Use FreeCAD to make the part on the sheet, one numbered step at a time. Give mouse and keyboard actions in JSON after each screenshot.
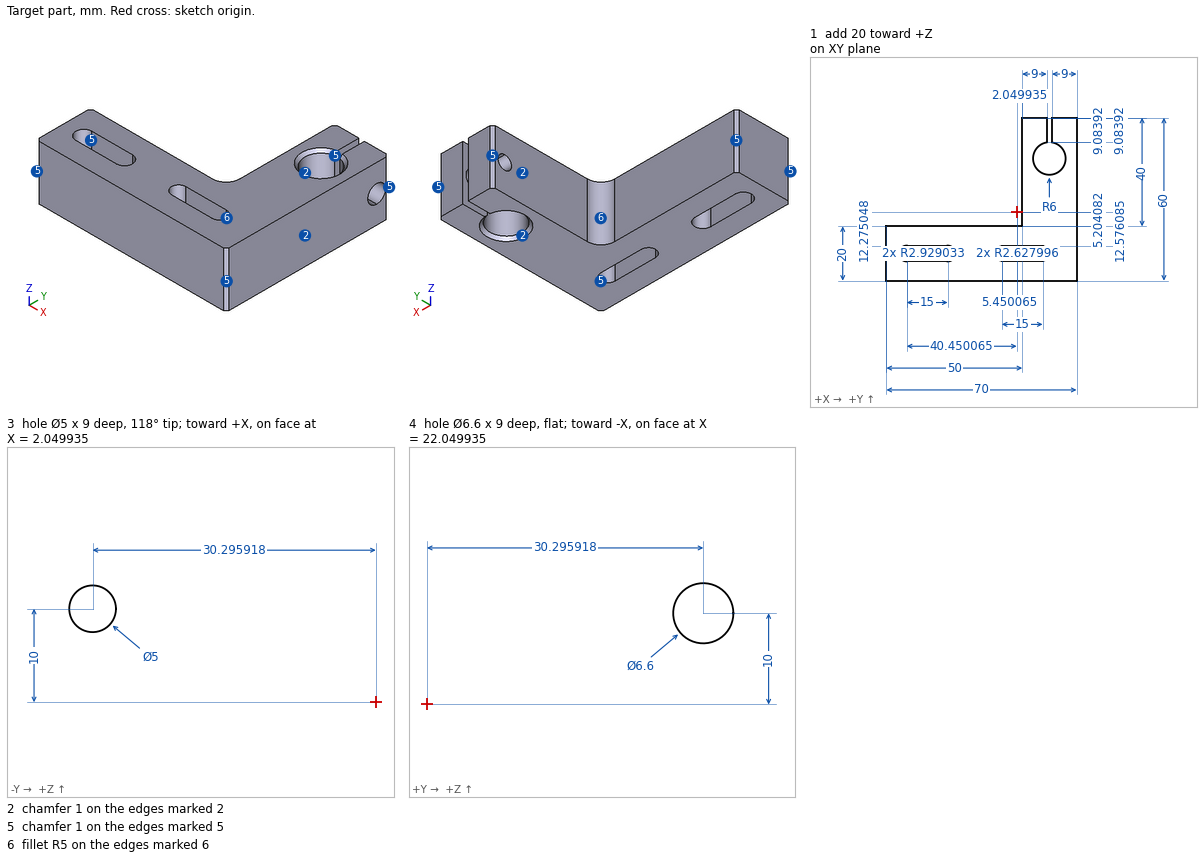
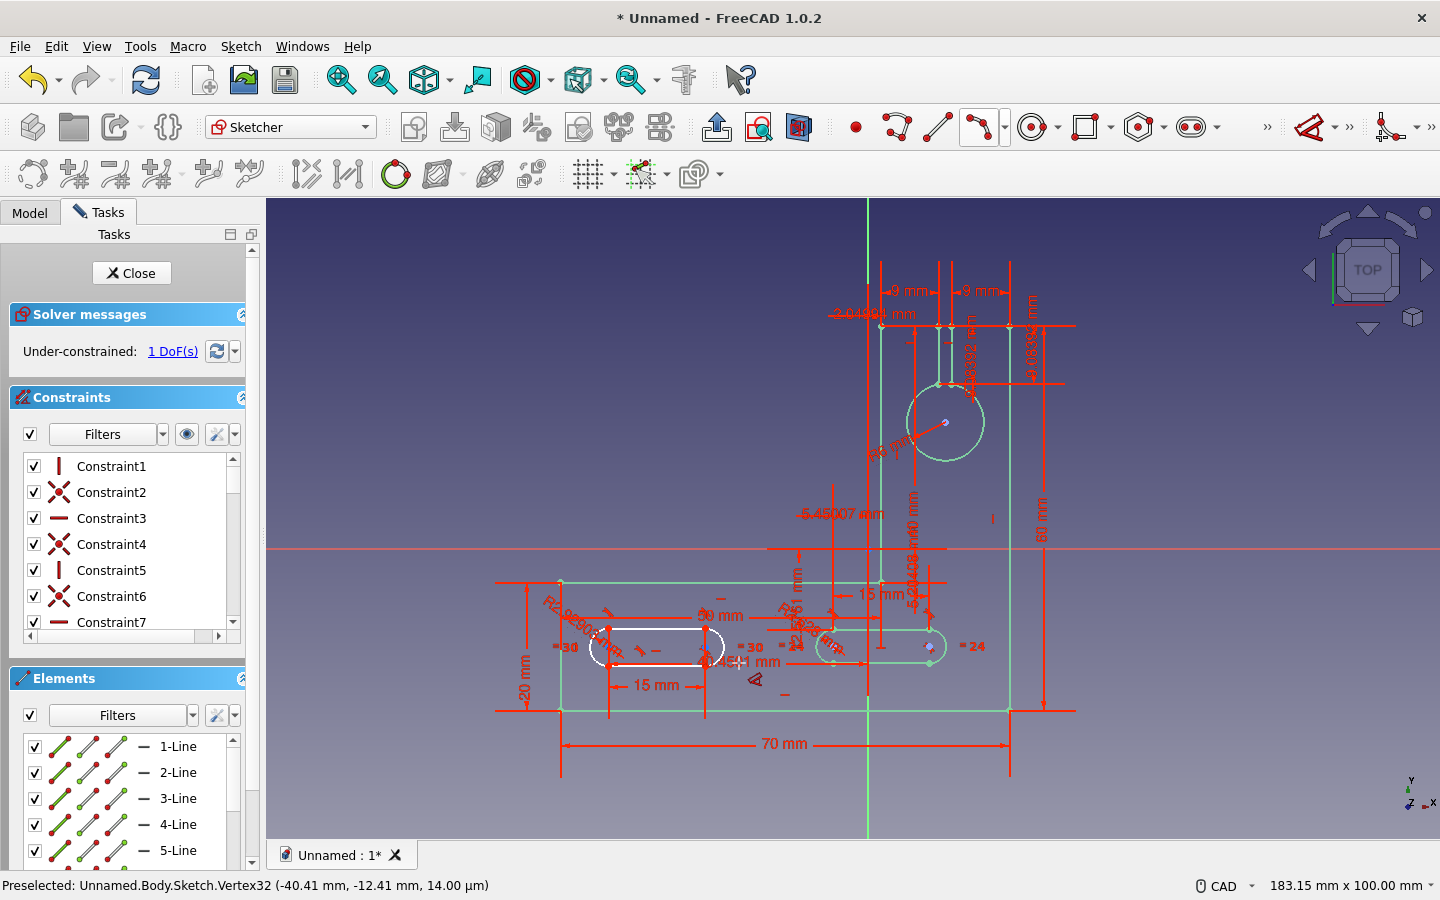
{"action": "left_click", "coordinate": [609, 629]}
{"action": "left_click", "coordinate": [575, 607]}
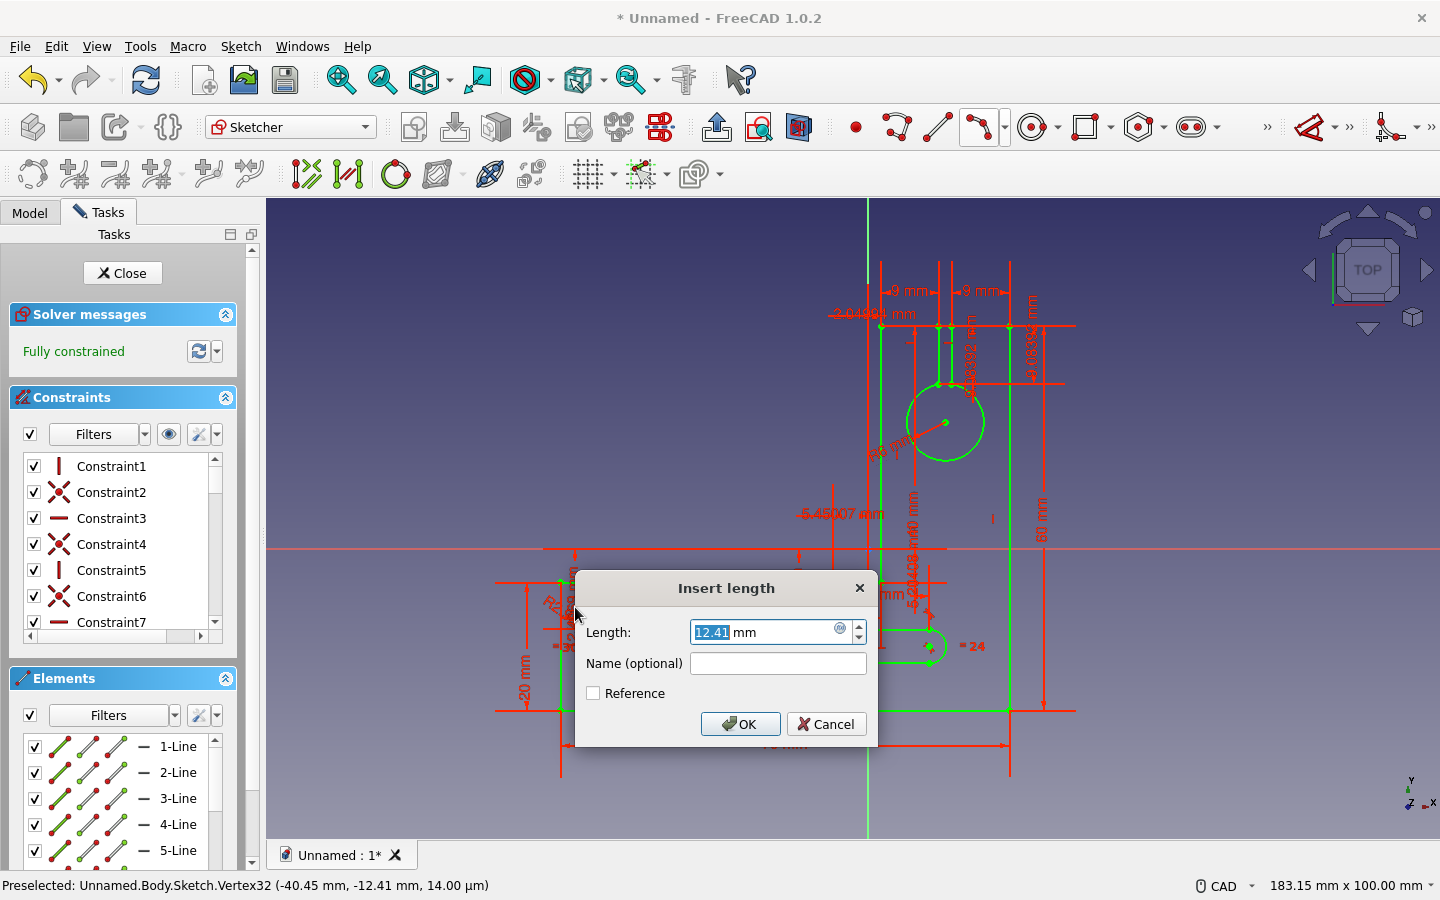
{"action": "type", "text": "12.275048"}
{"action": "key", "text": "Return"}
{"action": "key", "text": "Escape"}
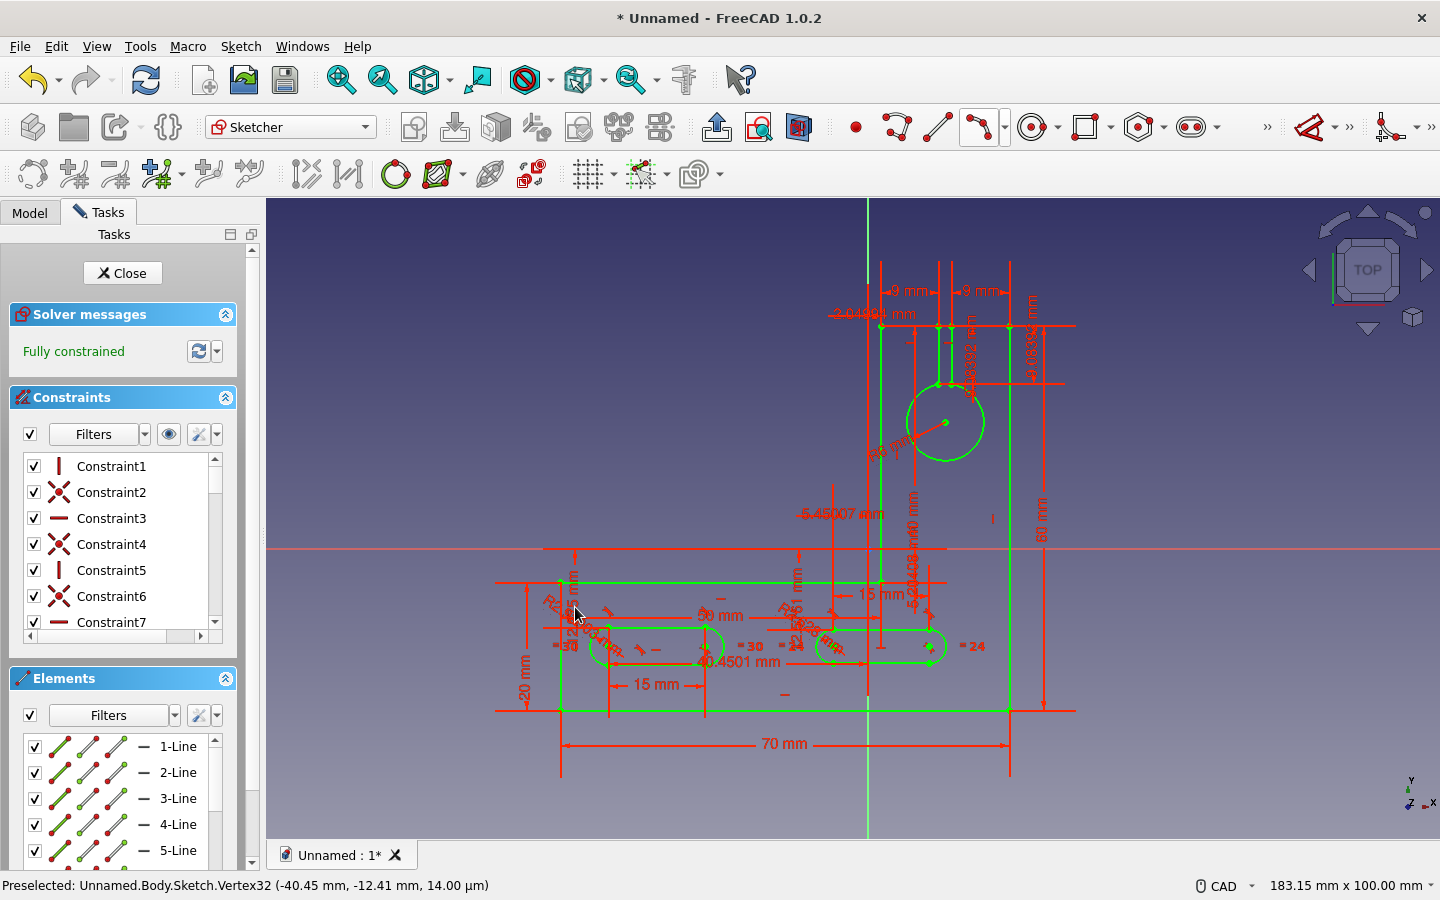
{"action": "left_click", "coordinate": [123, 273]}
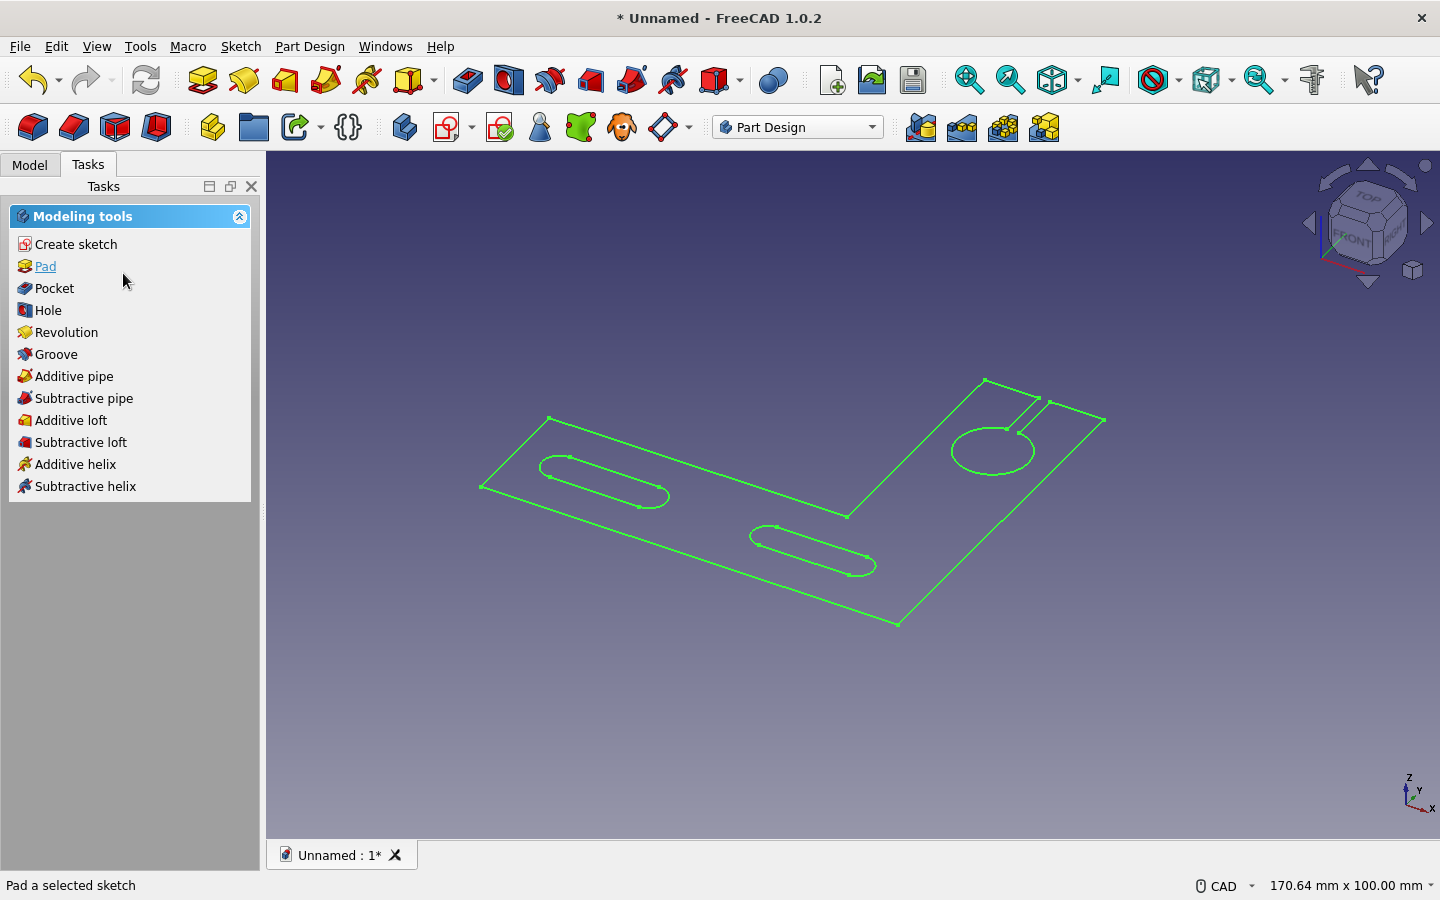
{"action": "left_click", "coordinate": [203, 80]}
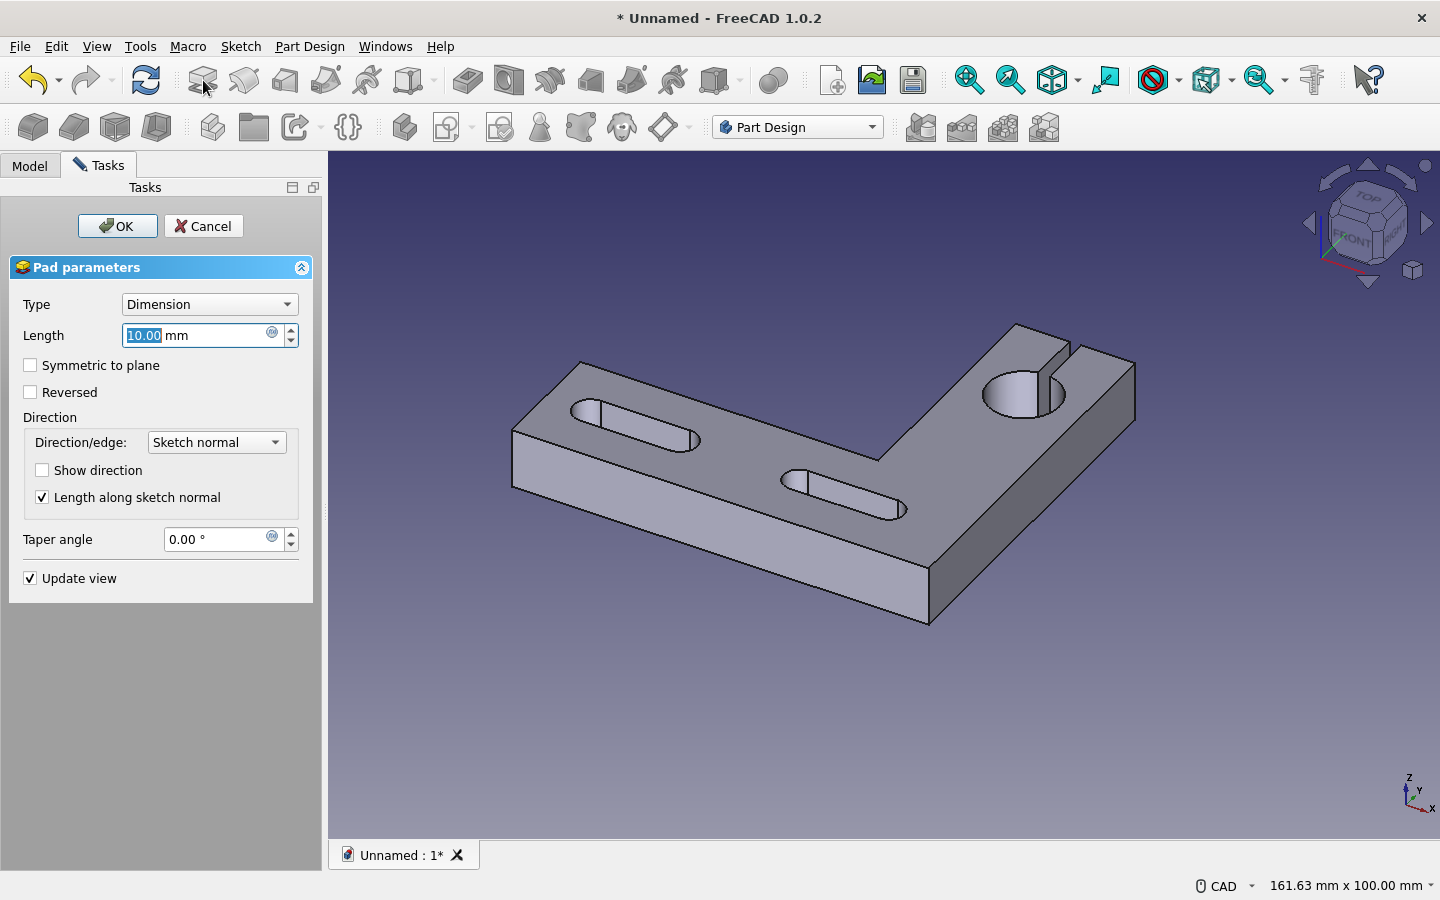
{"action": "type", "text": "20"}
{"action": "key", "text": "Tab"}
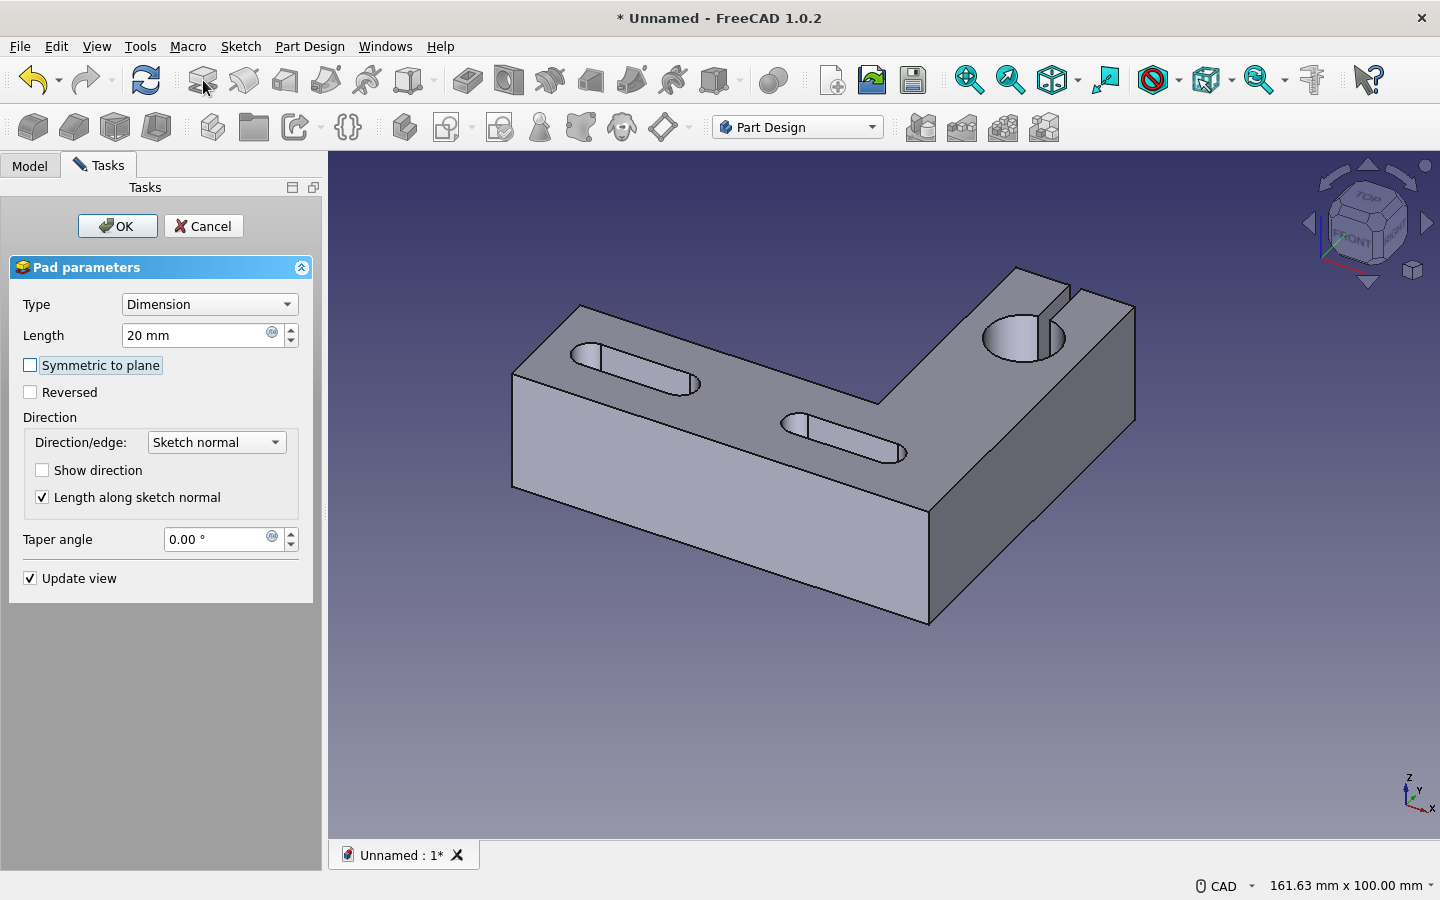
{"action": "left_click", "coordinate": [118, 226]}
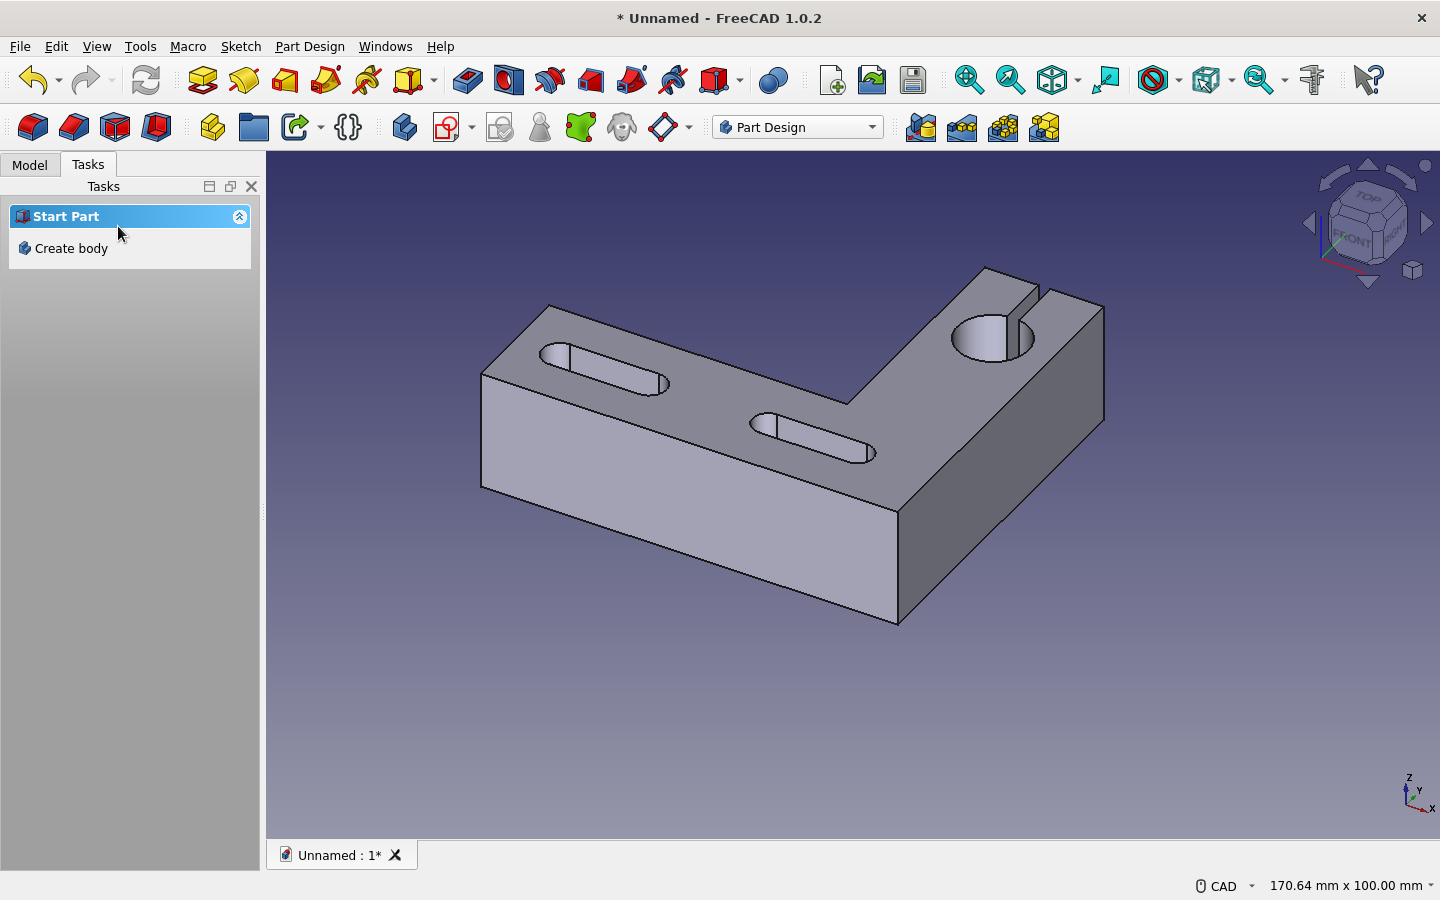
{"action": "left_click", "coordinate": [952, 334]}